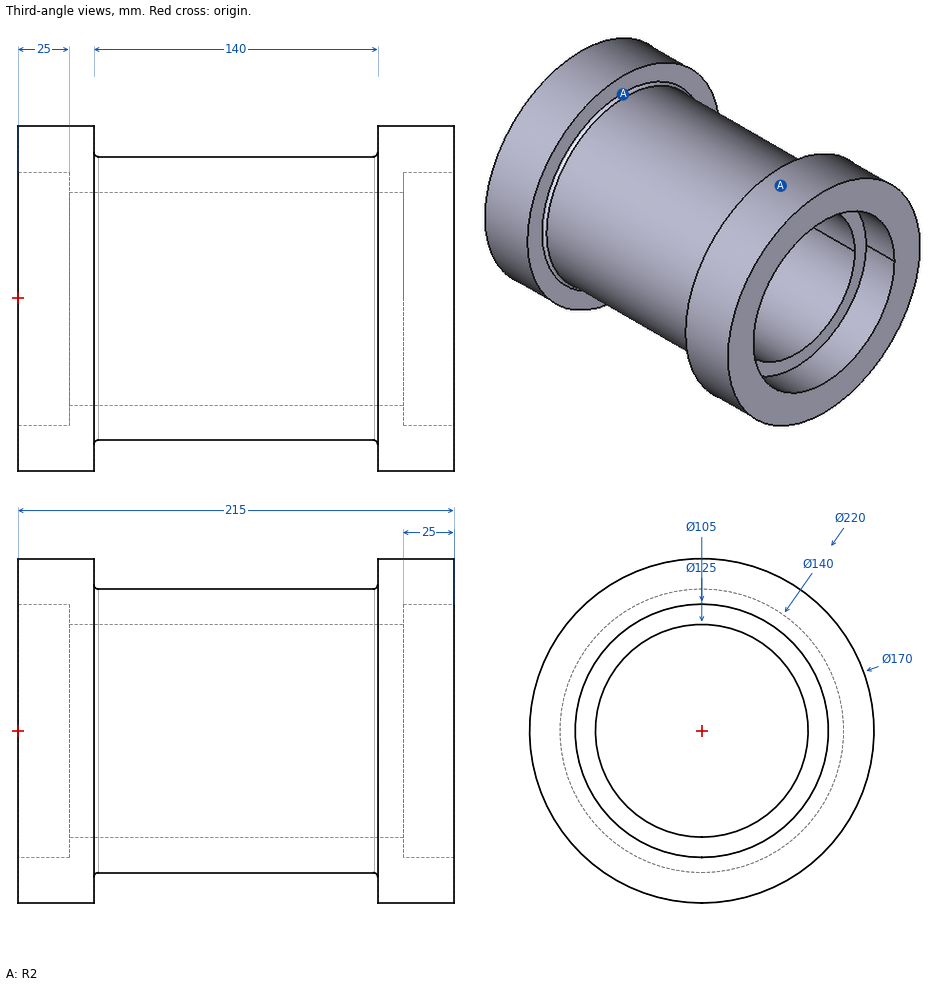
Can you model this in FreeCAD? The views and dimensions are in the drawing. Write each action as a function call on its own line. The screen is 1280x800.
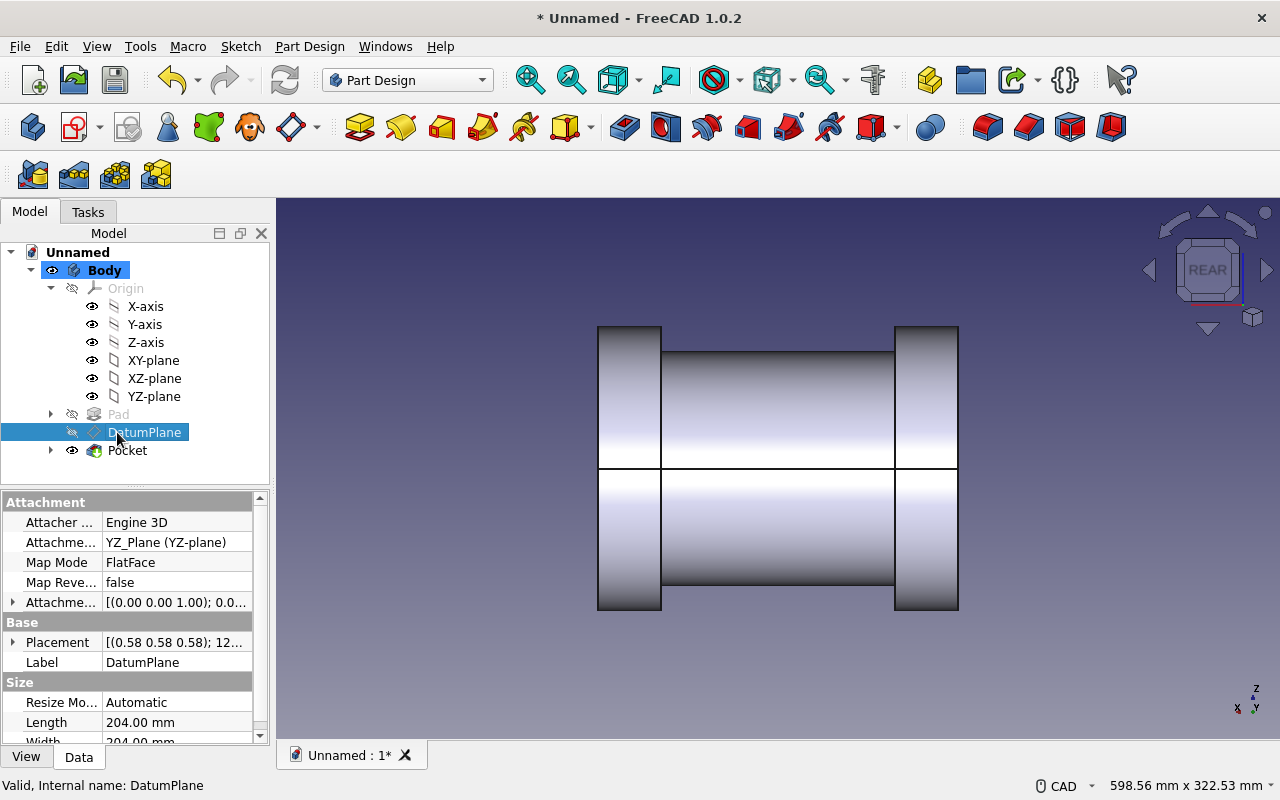
key(6)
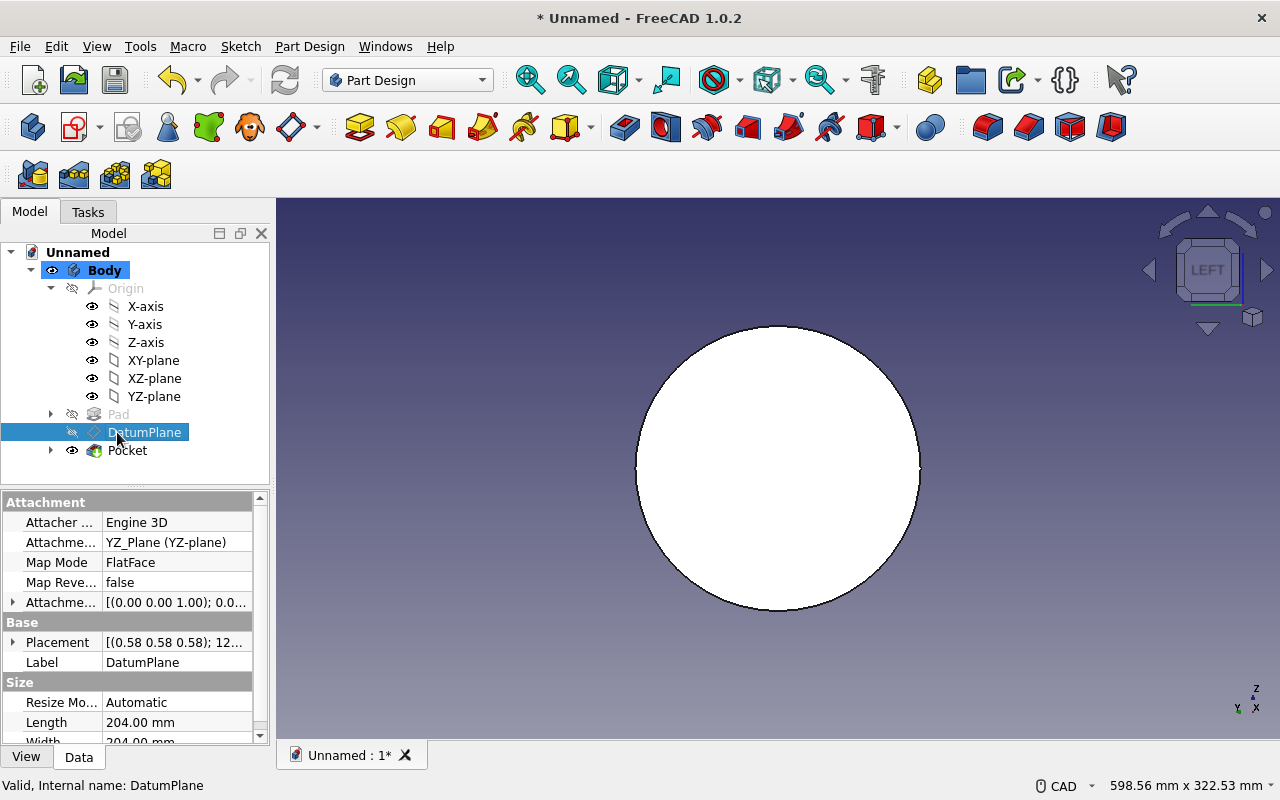
key(v)
key(3)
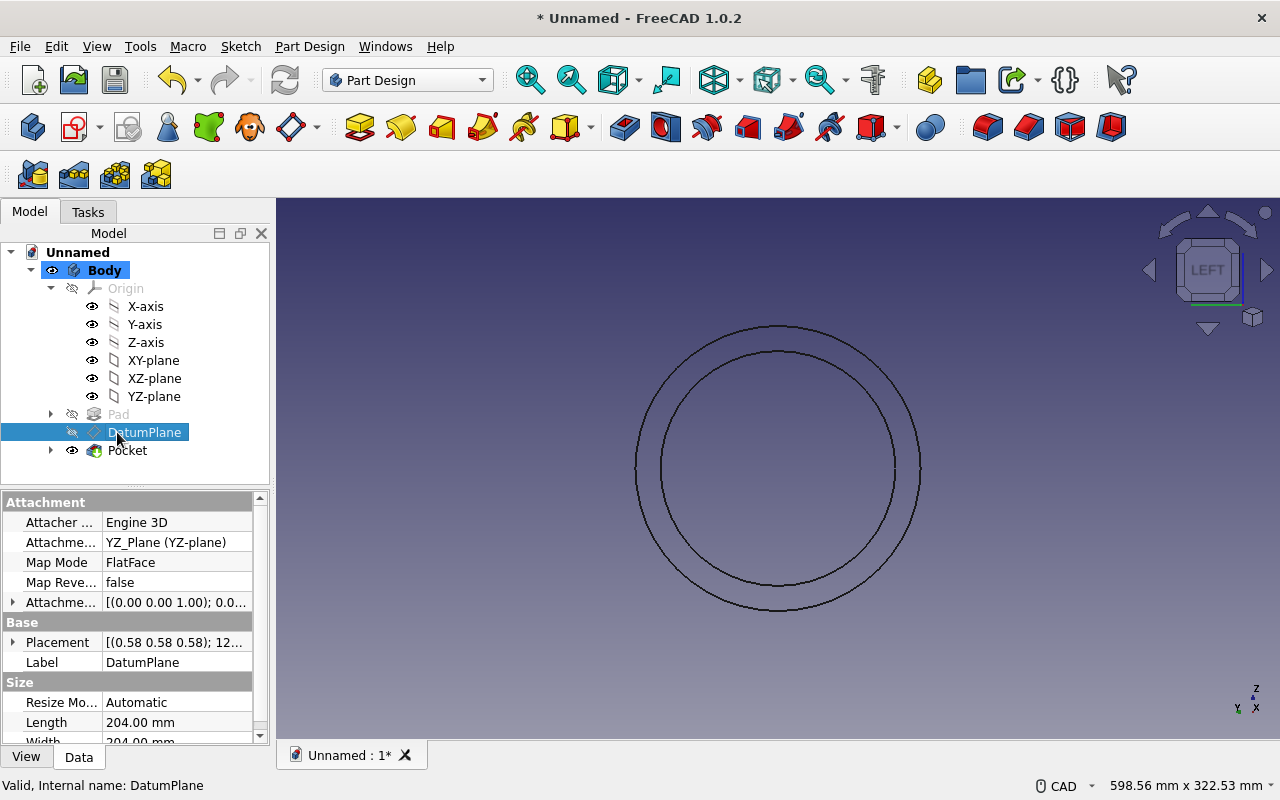
key(0)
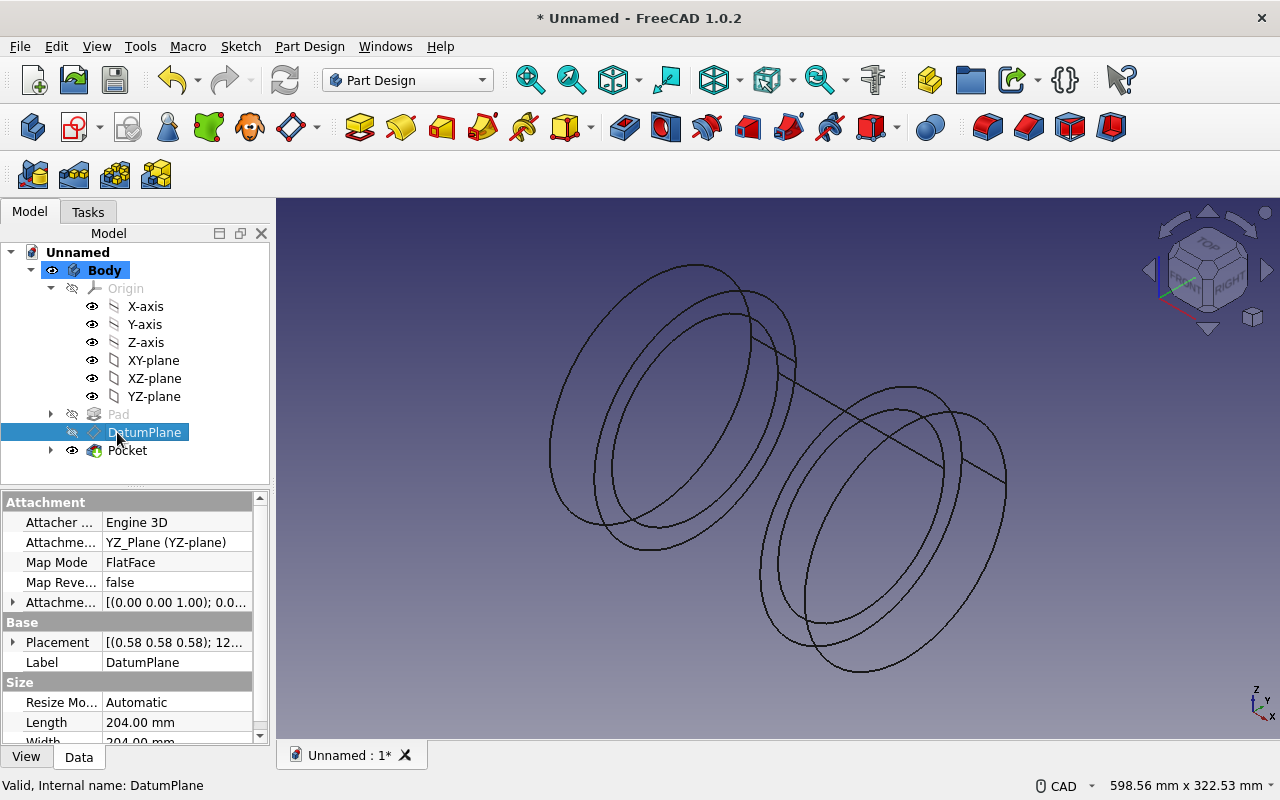
click(612, 468)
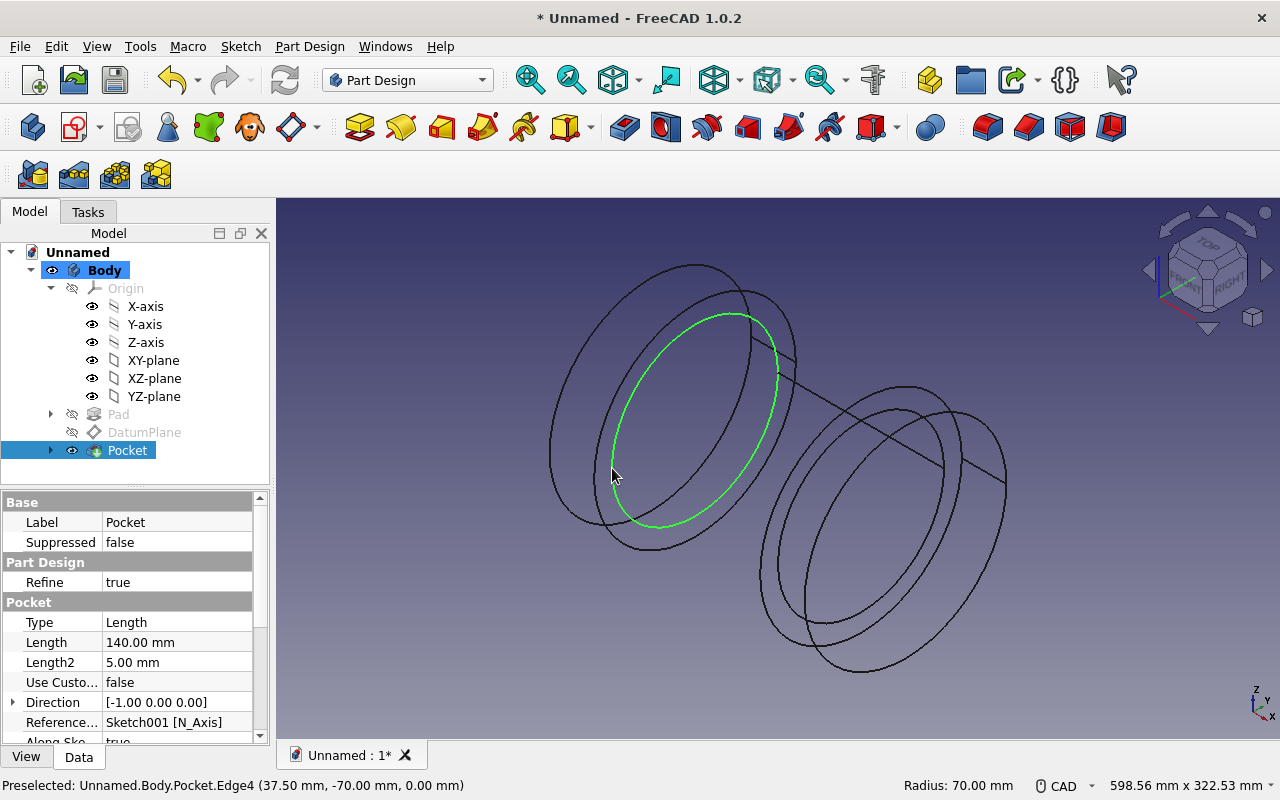
click(778, 563, ctrl)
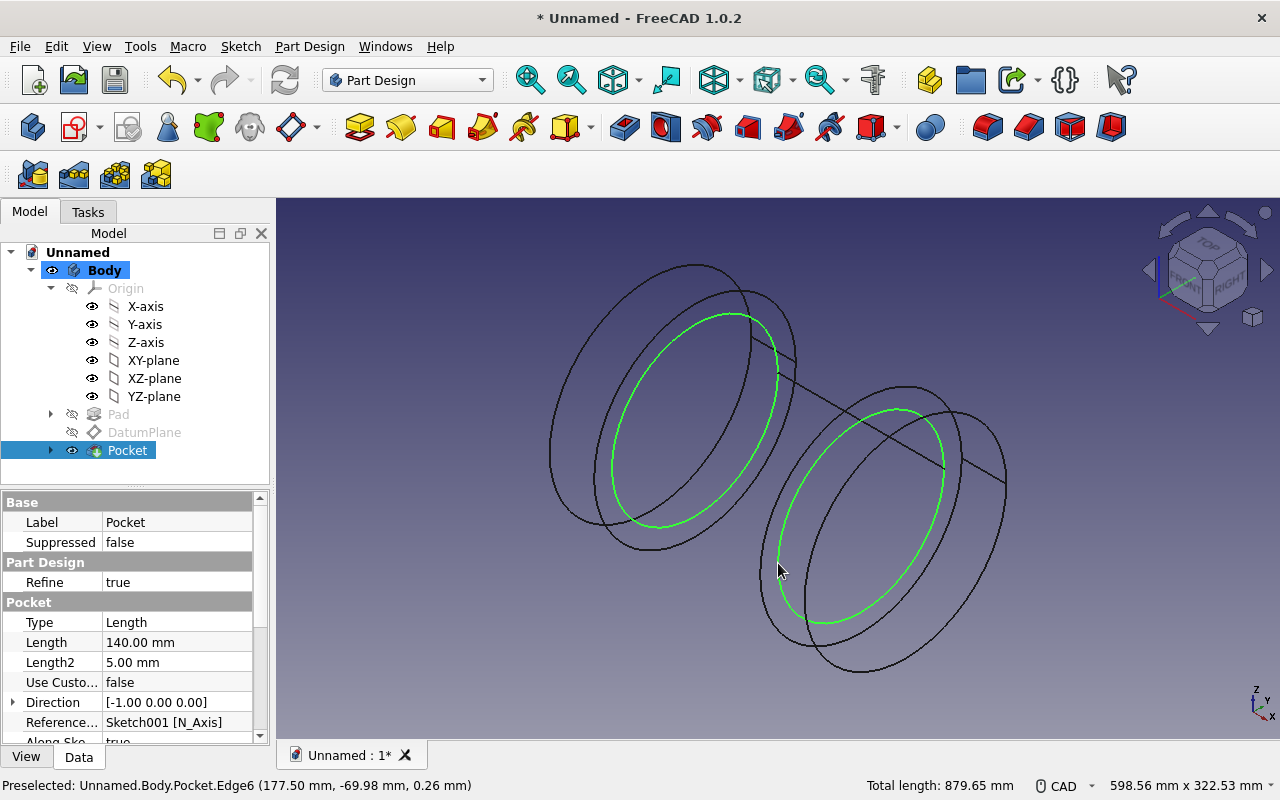
key(v)
key(1)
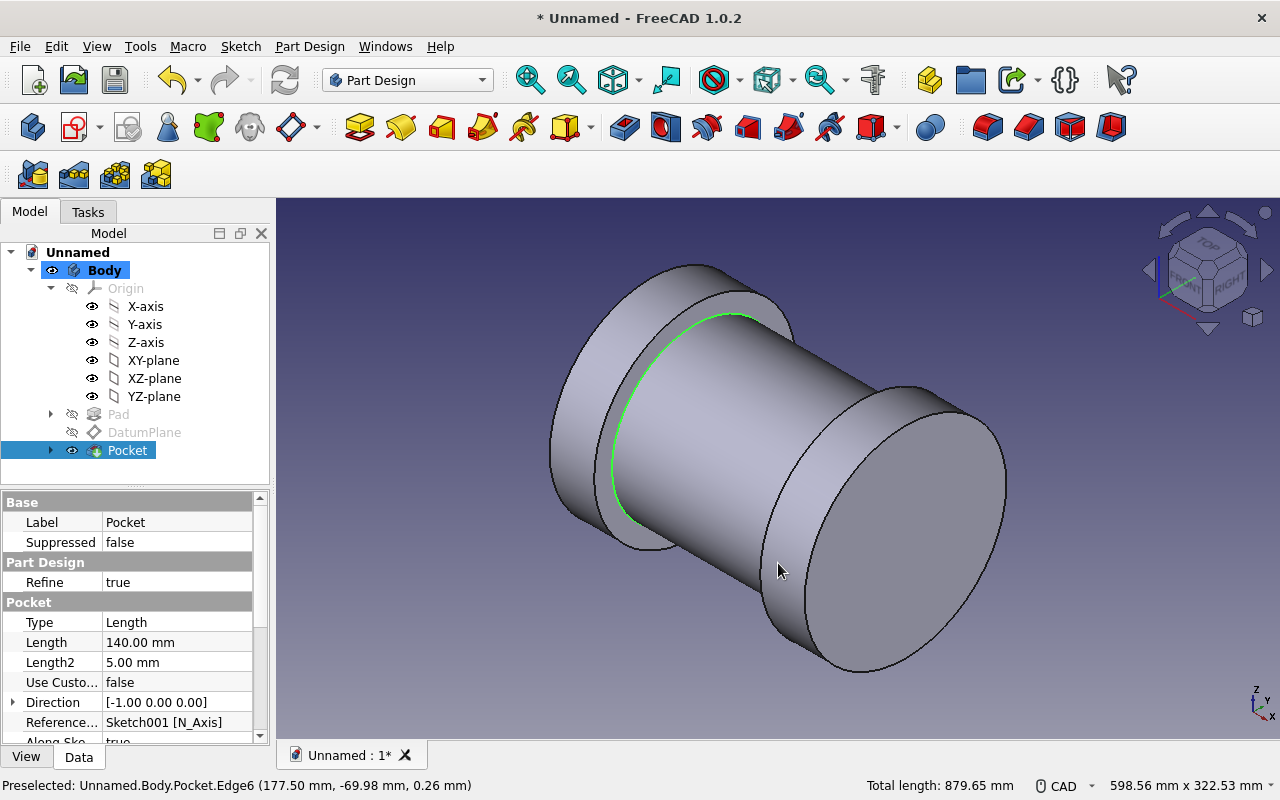
click(988, 128)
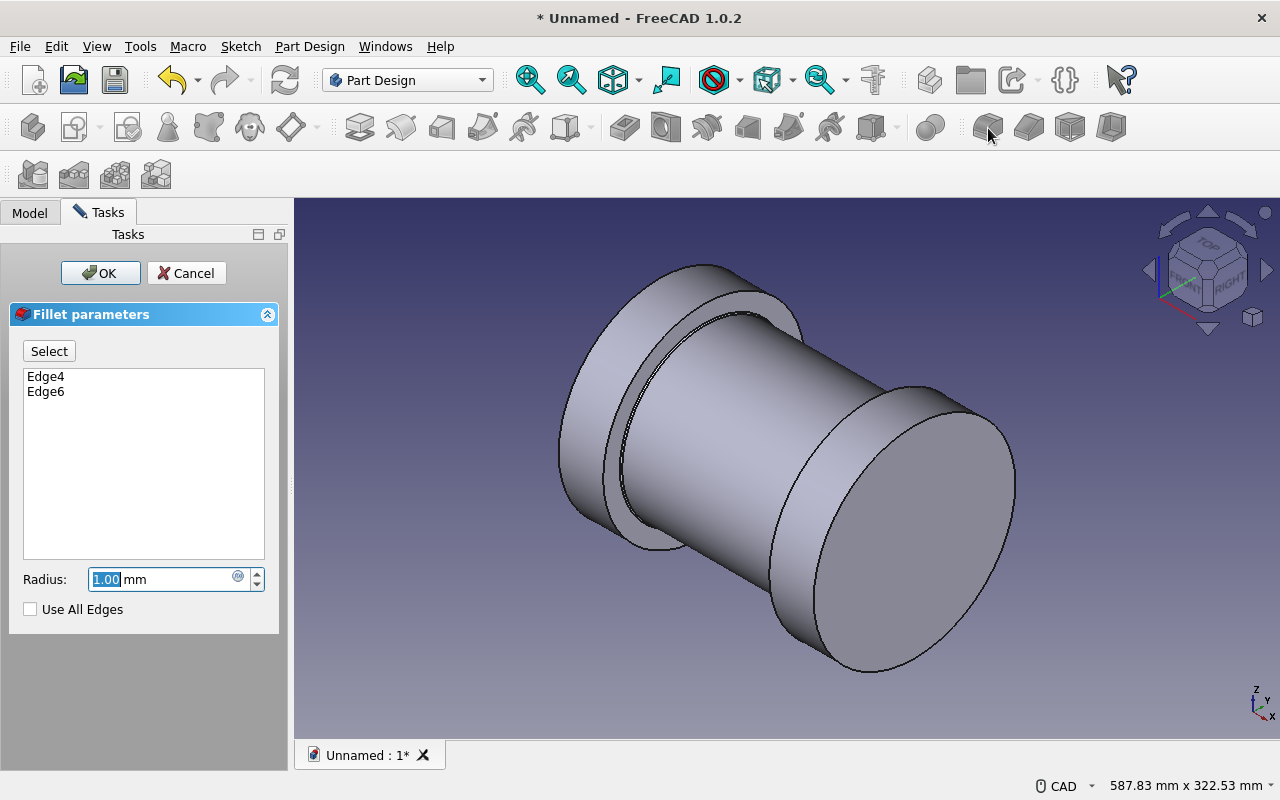
text(2)
key(Tab)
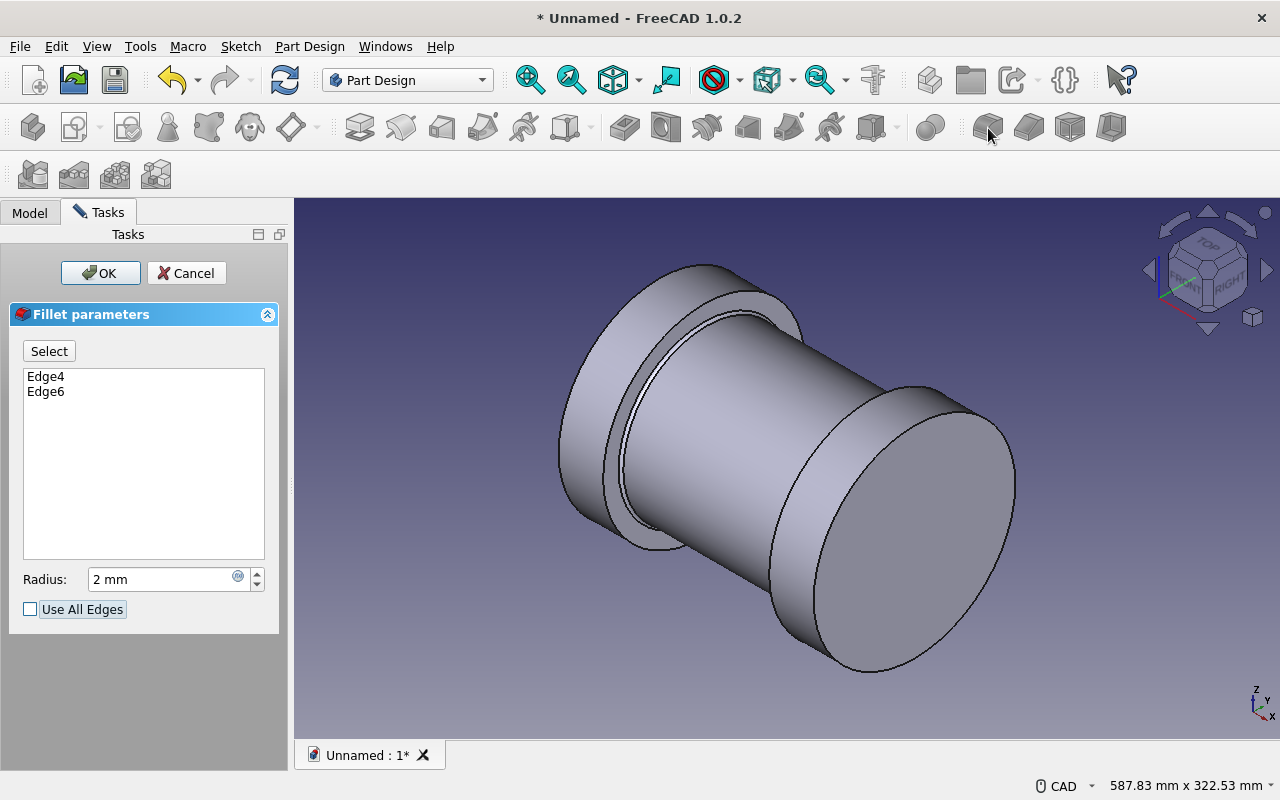
click(101, 273)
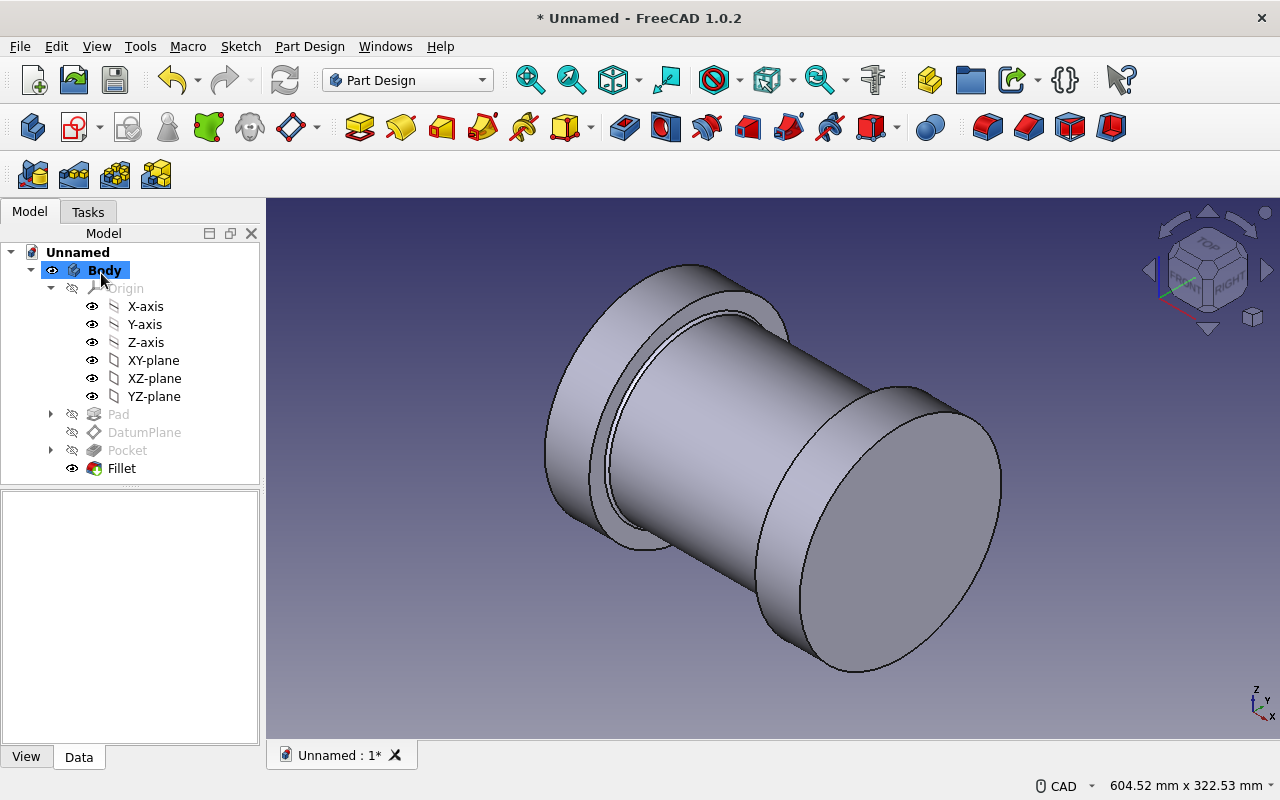
click(901, 541)